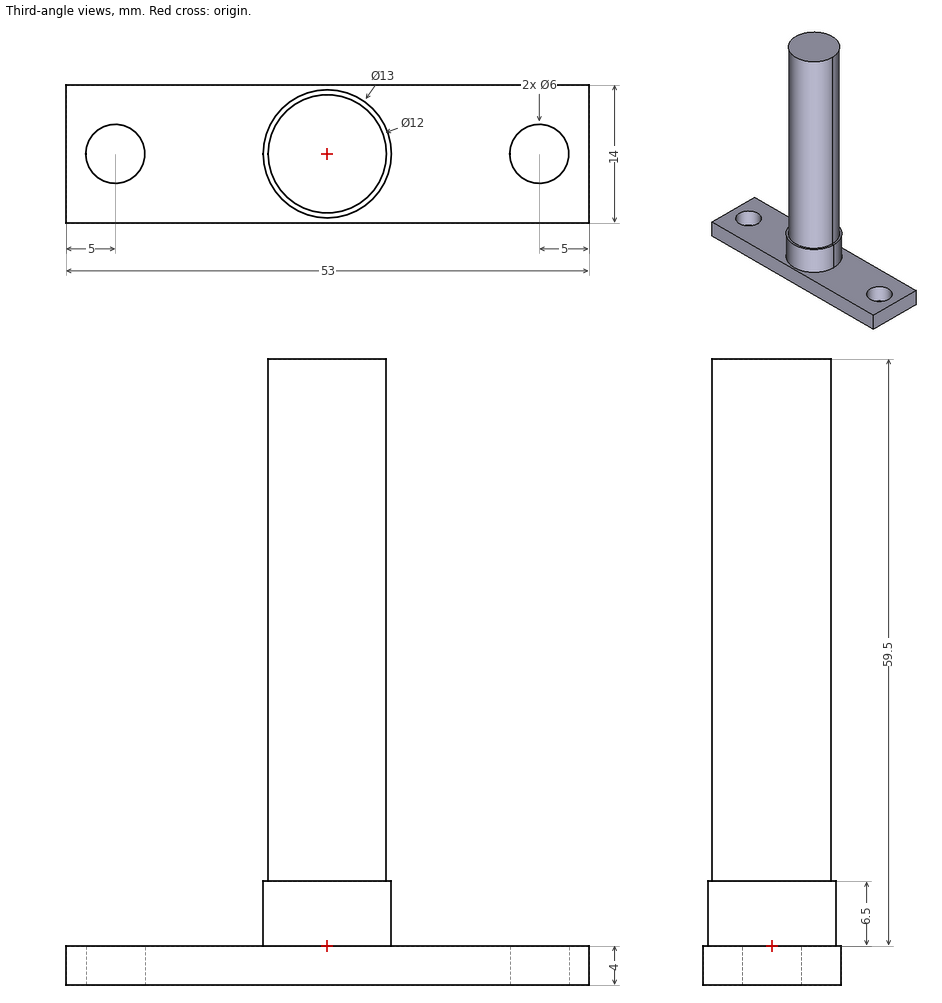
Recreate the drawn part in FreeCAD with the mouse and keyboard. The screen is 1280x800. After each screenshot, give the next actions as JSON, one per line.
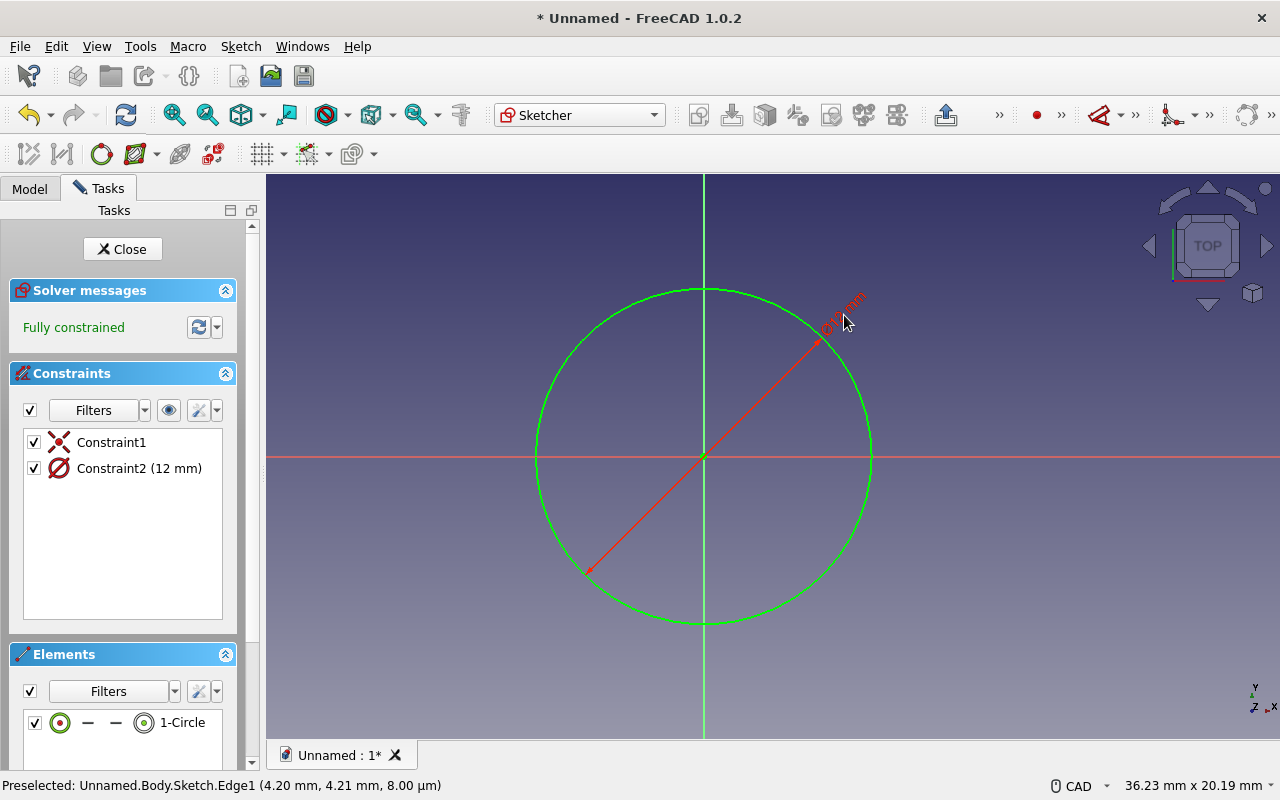
{"action": "left_click", "coordinate": [123, 249]}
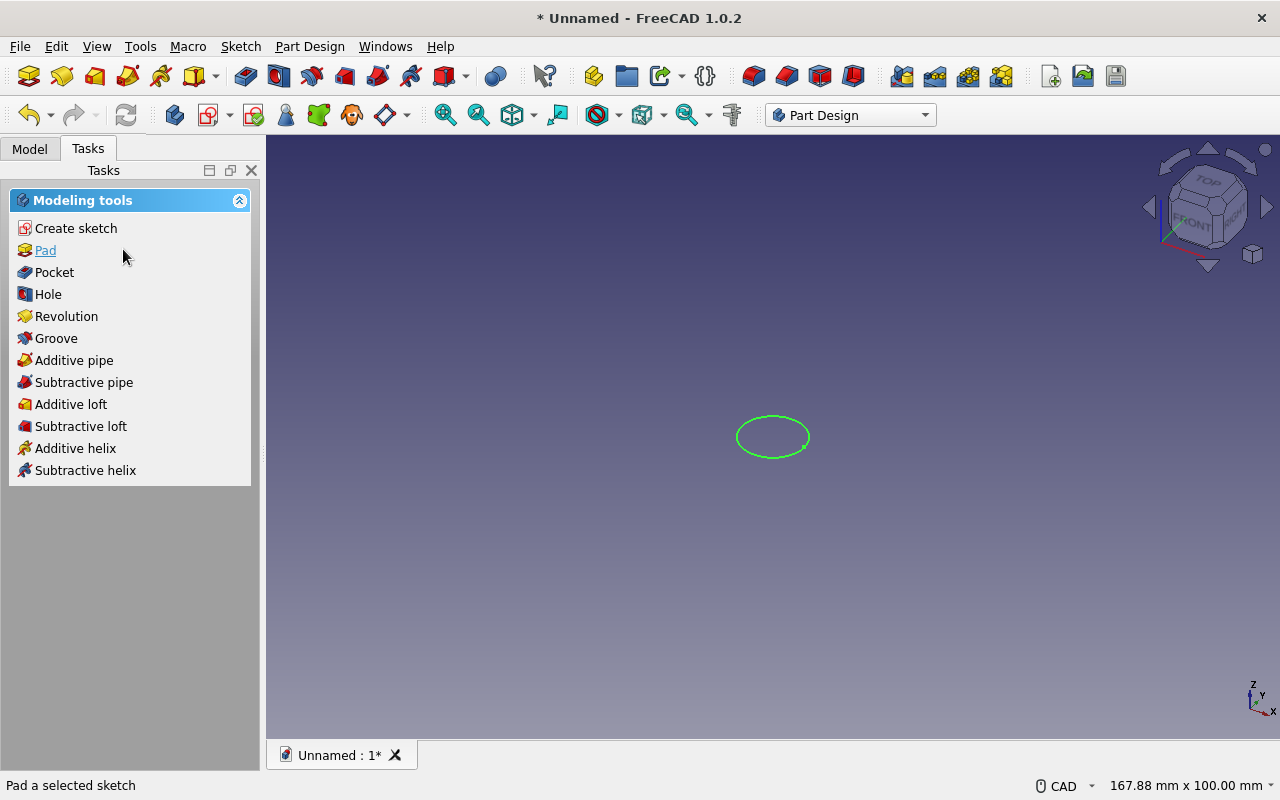
{"action": "left_click", "coordinate": [29, 76]}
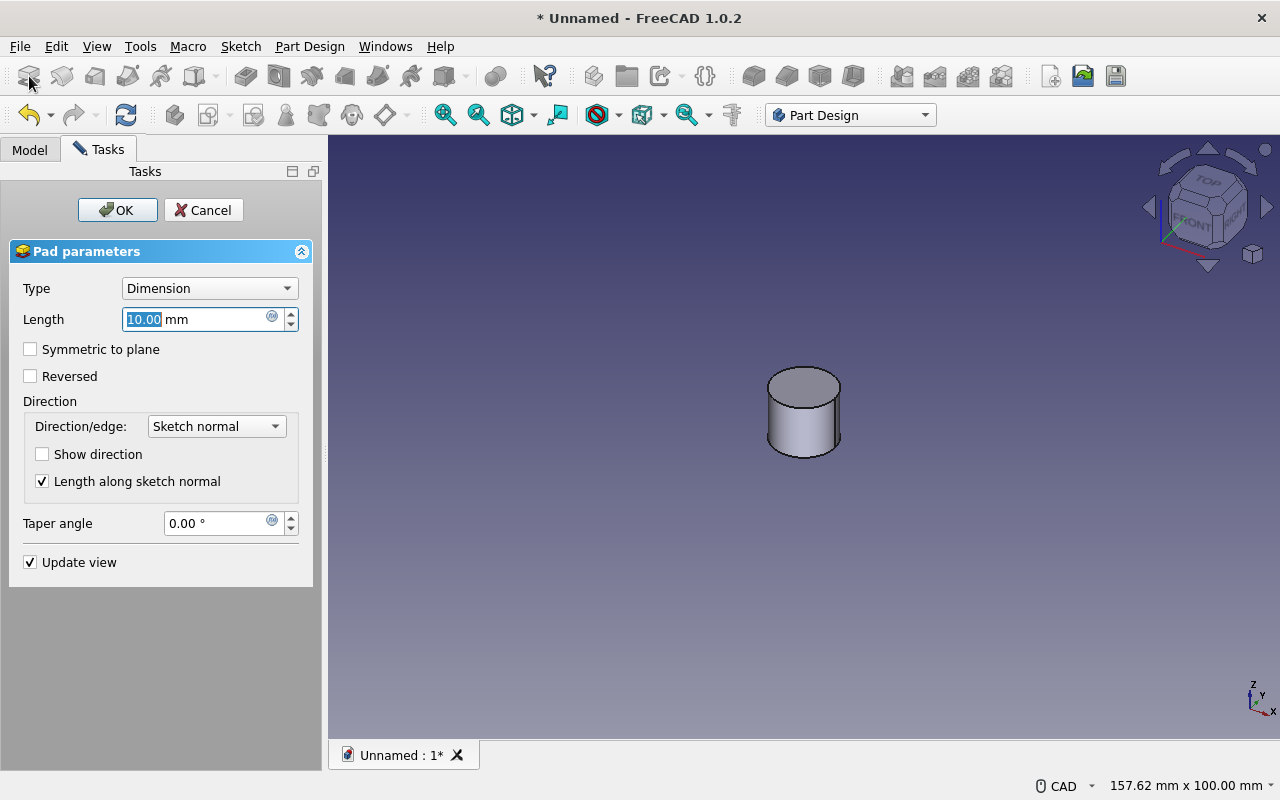
{"action": "type", "text": "59.5"}
{"action": "key", "text": "Tab"}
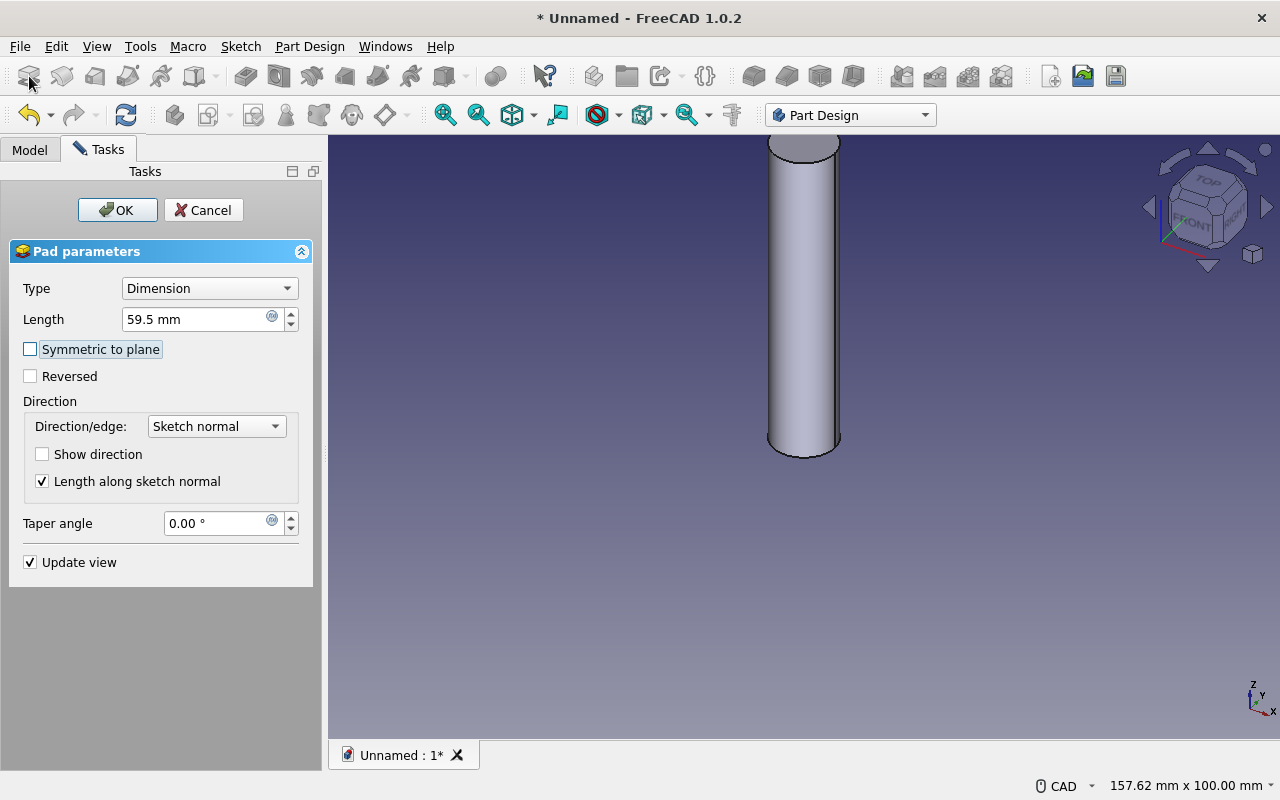
{"action": "left_click", "coordinate": [118, 210]}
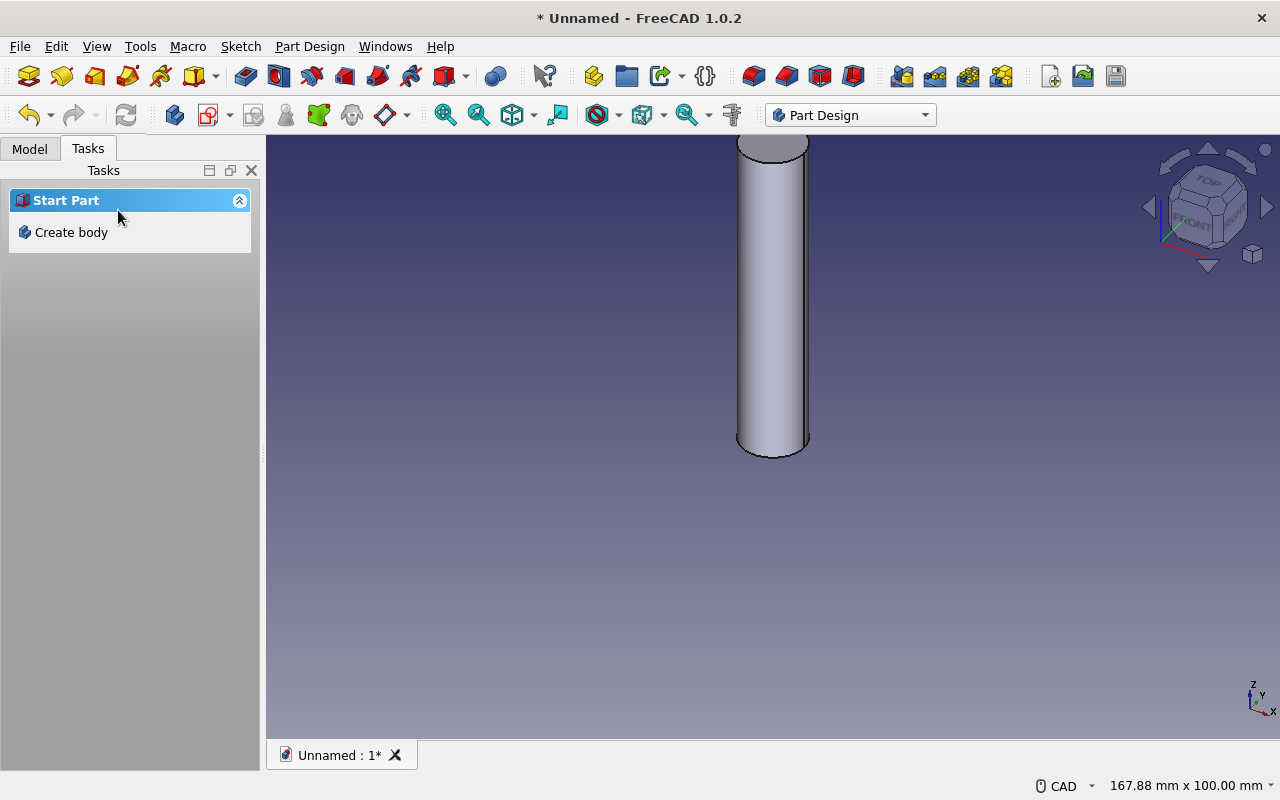
{"action": "left_click", "coordinate": [446, 116]}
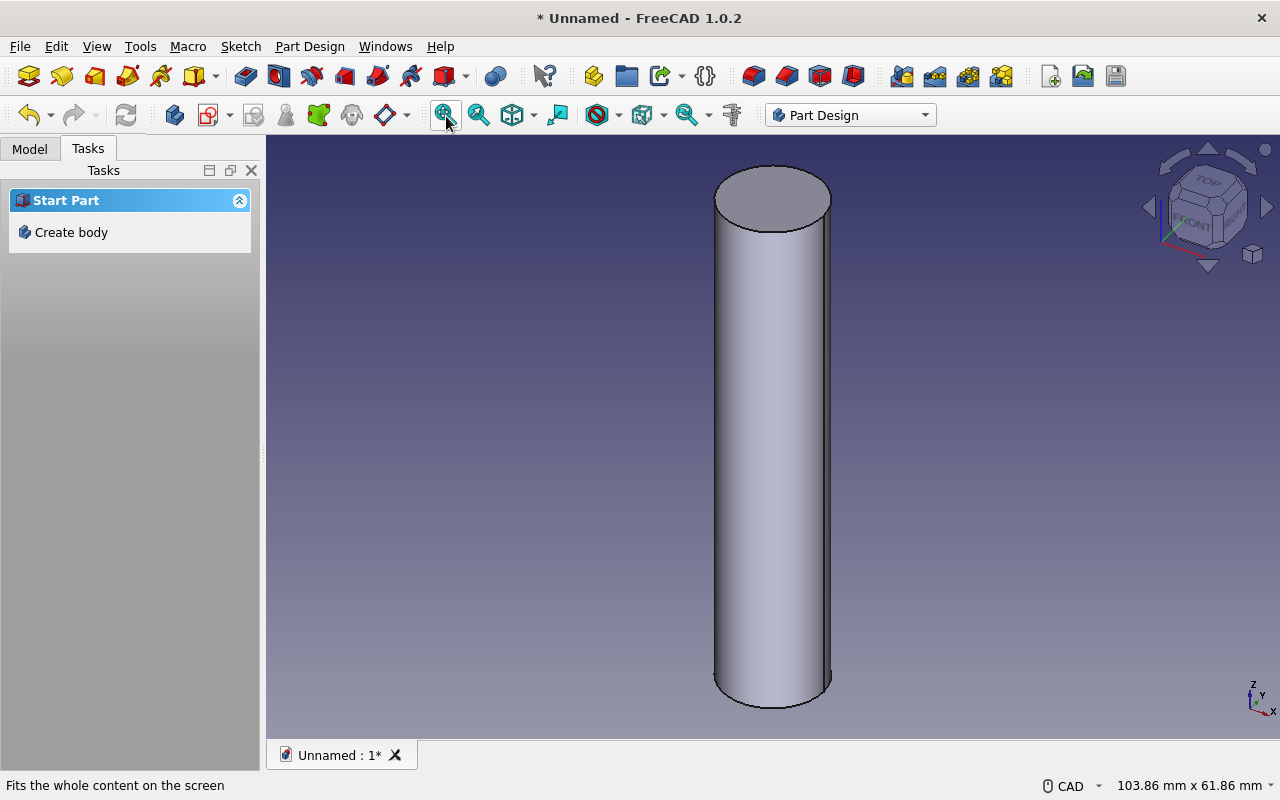
{"action": "left_click", "coordinate": [208, 116]}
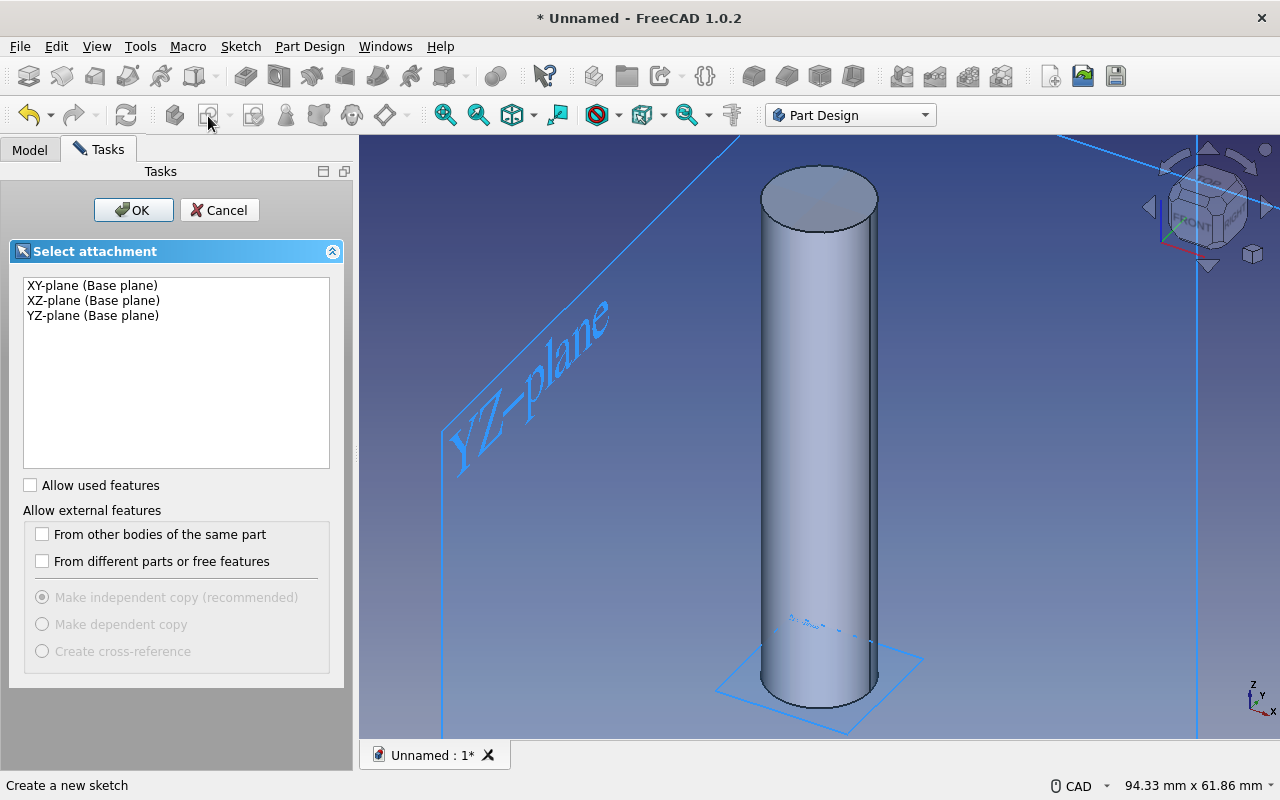
{"action": "left_click", "coordinate": [84, 286]}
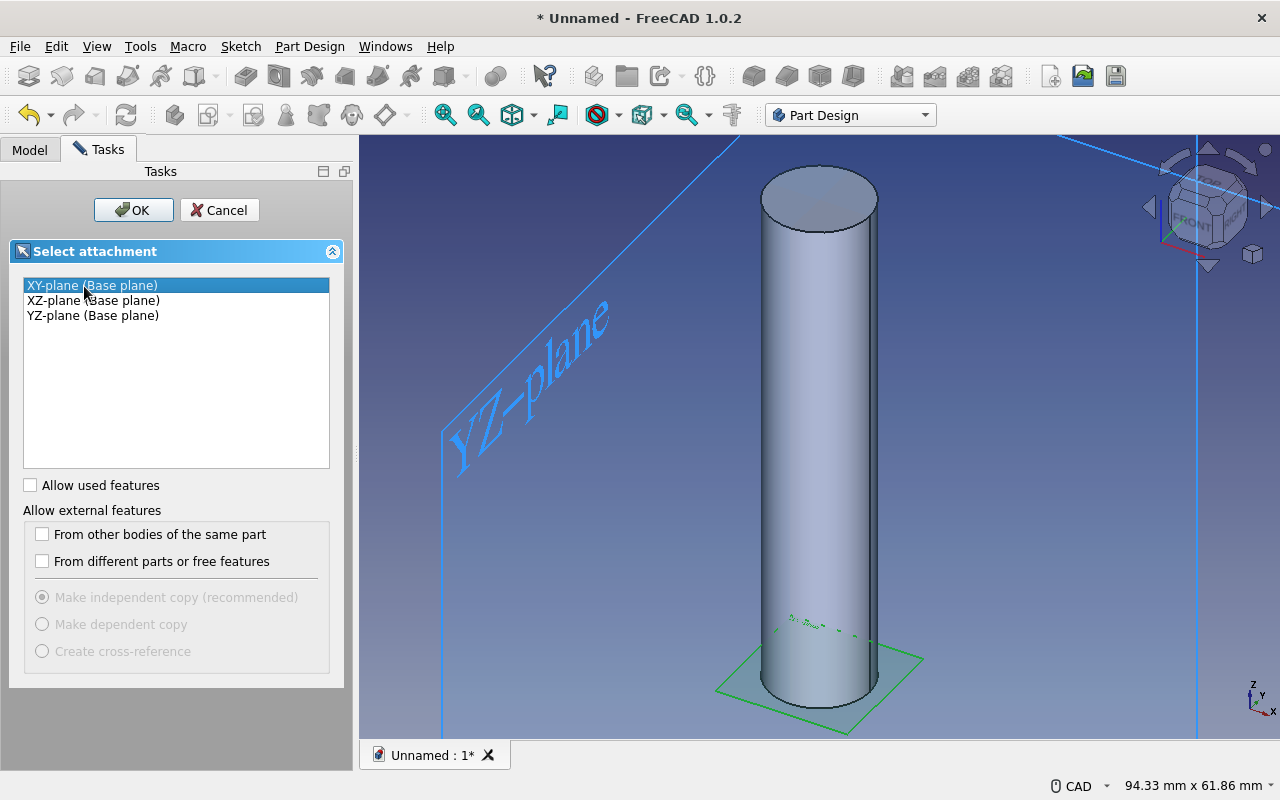
{"action": "left_click", "coordinate": [134, 210]}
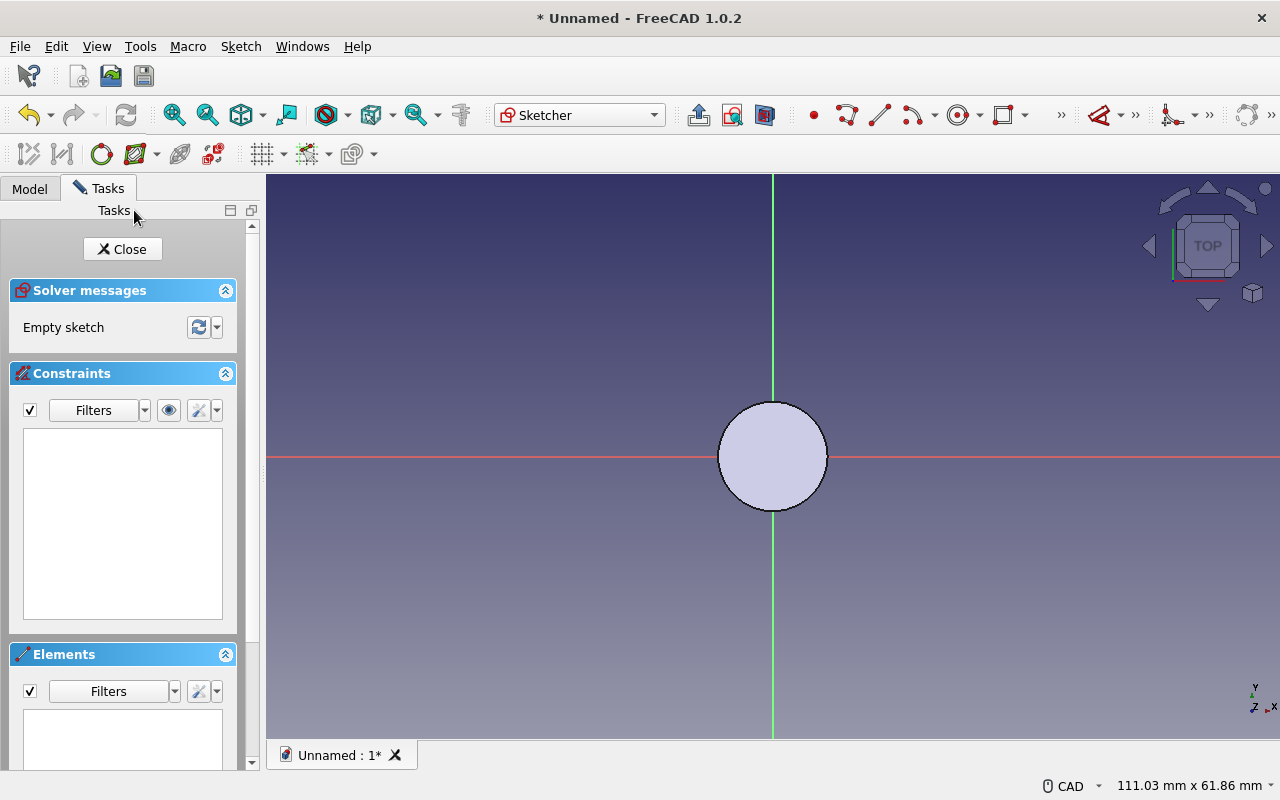
{"action": "key", "text": "q s"}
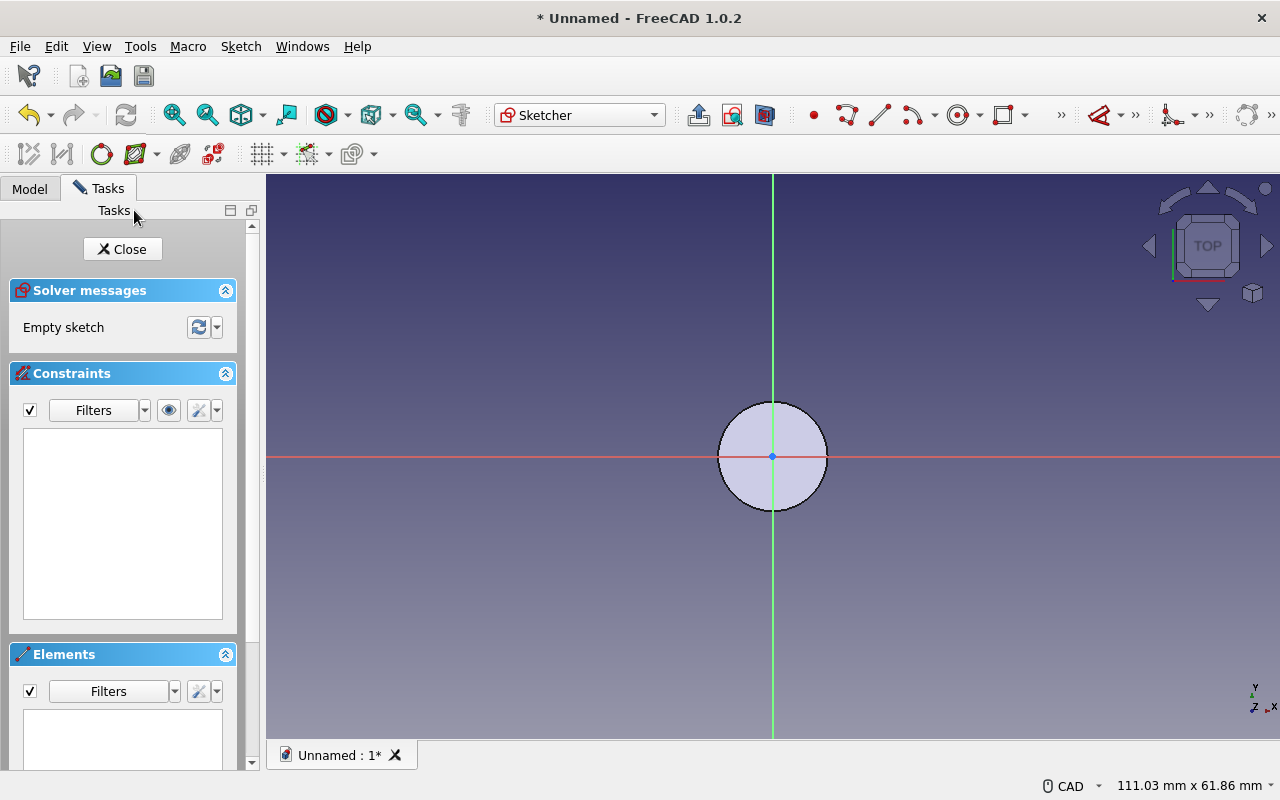
{"action": "key", "text": "g v"}